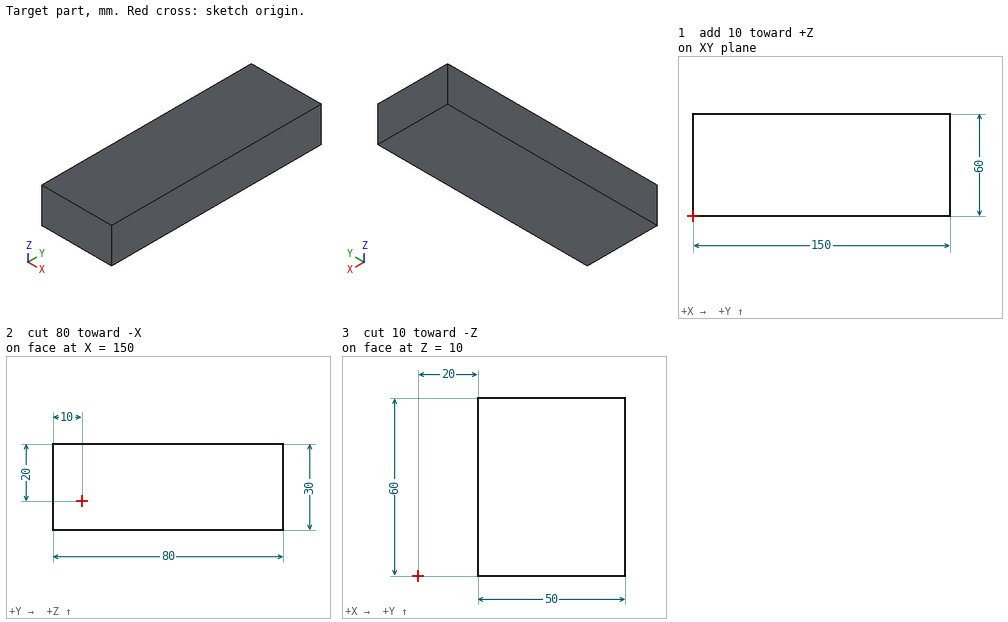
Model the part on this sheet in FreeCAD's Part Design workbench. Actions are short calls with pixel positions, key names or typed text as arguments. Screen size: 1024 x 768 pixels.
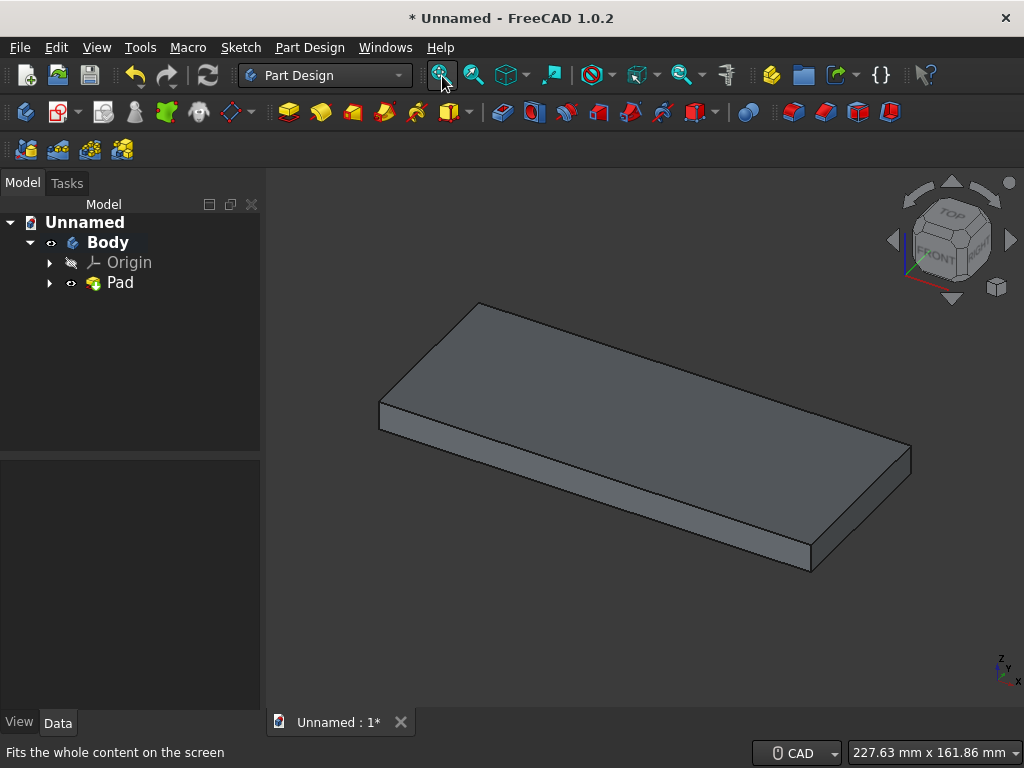
click(890, 480)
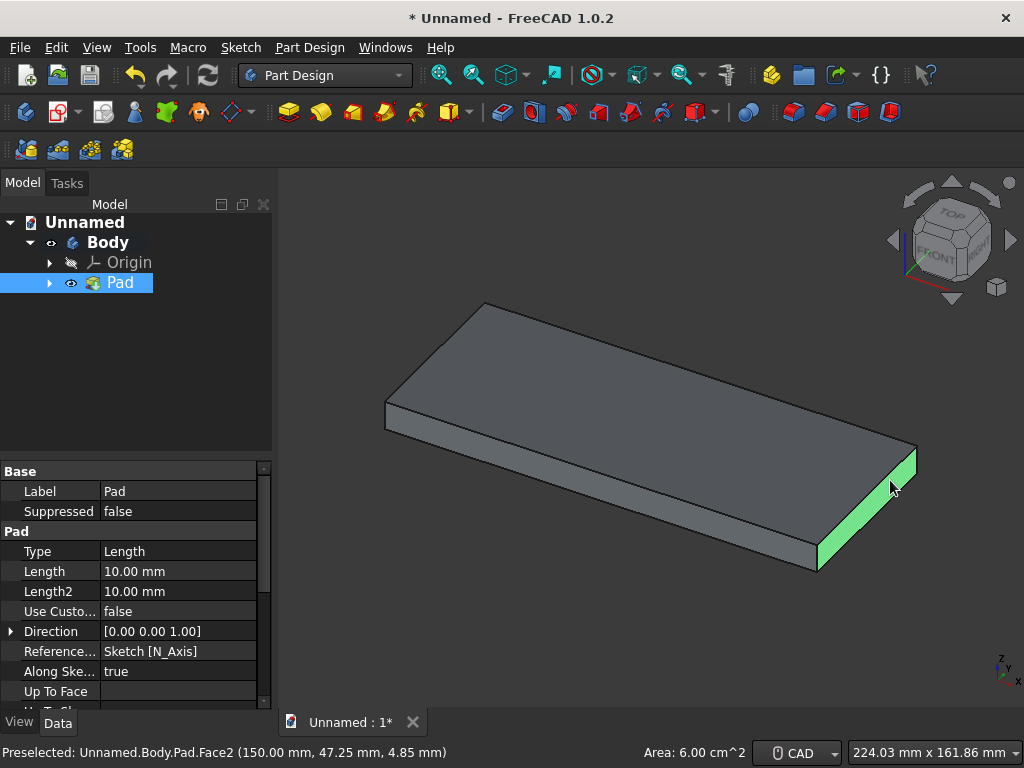
click(58, 112)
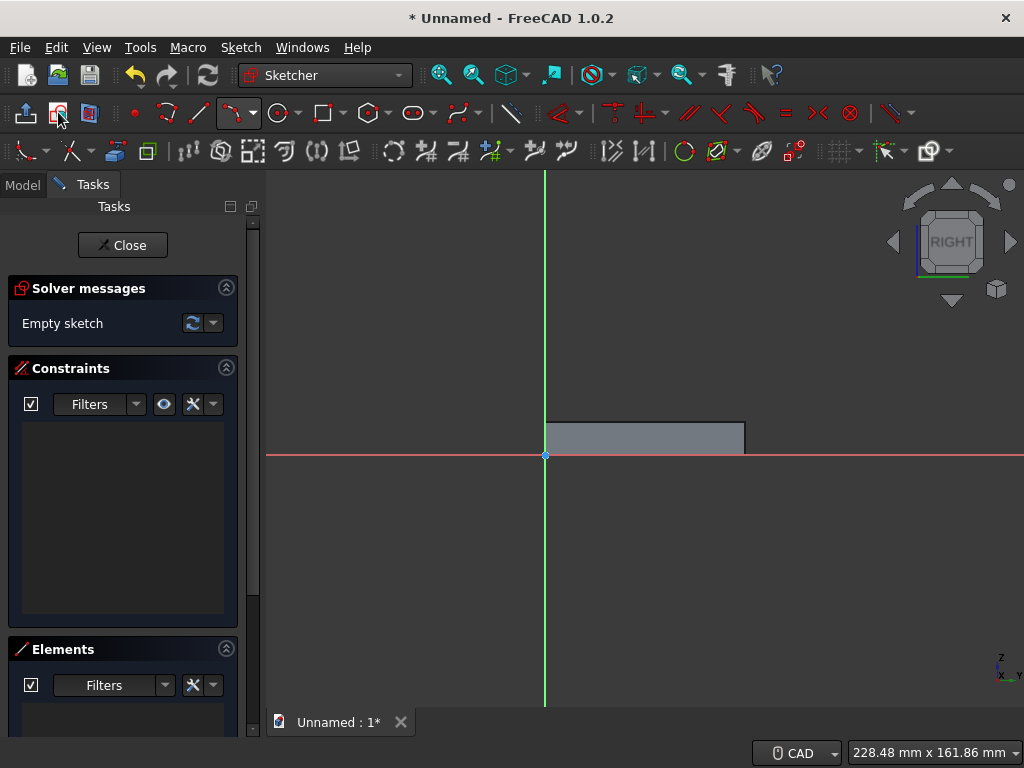
scroll(784, 439, up, 2)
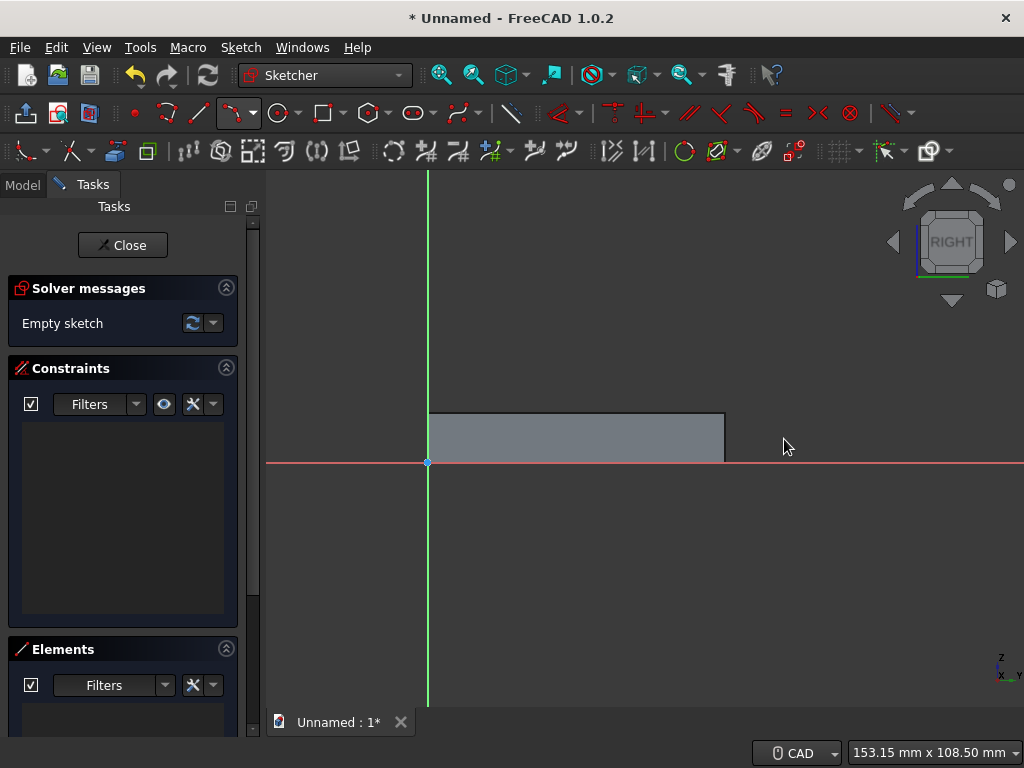
click(324, 114)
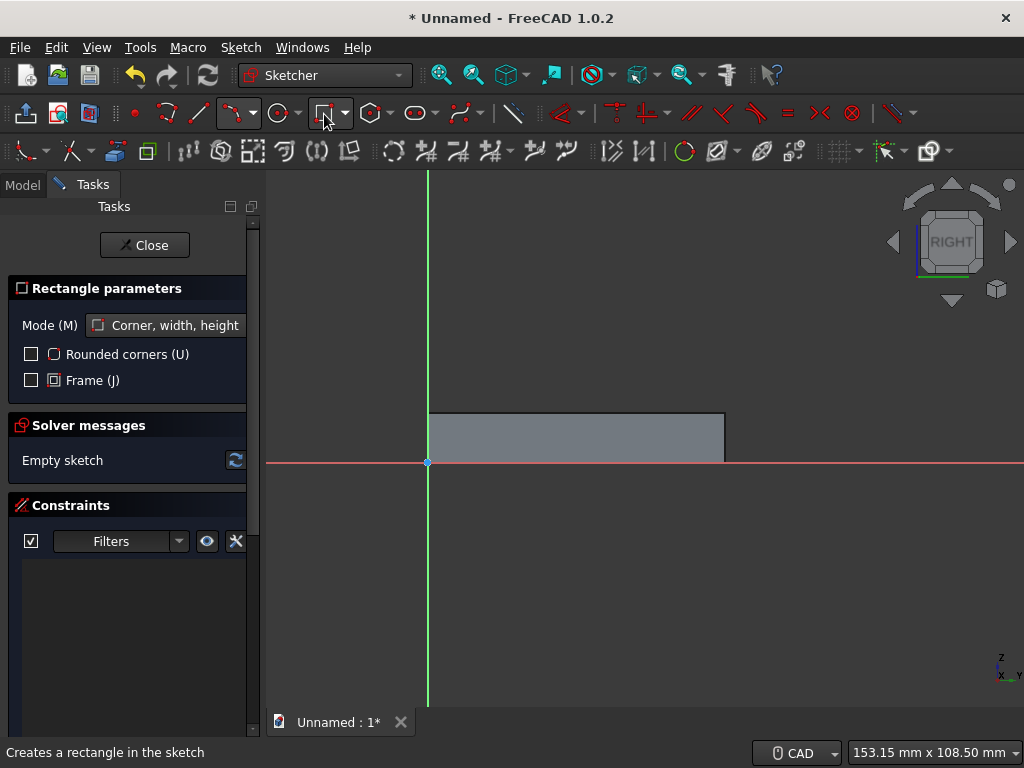
click(378, 364)
move(774, 512)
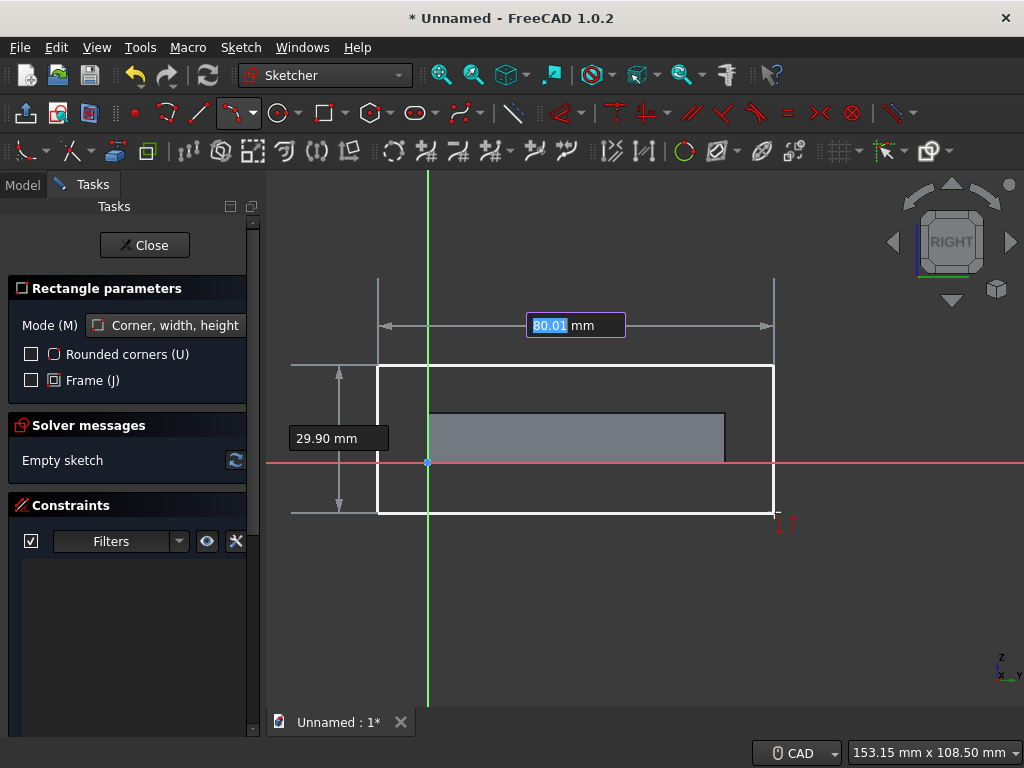
text(80)
key(Tab)
text(30)
key(Return)
key(Escape)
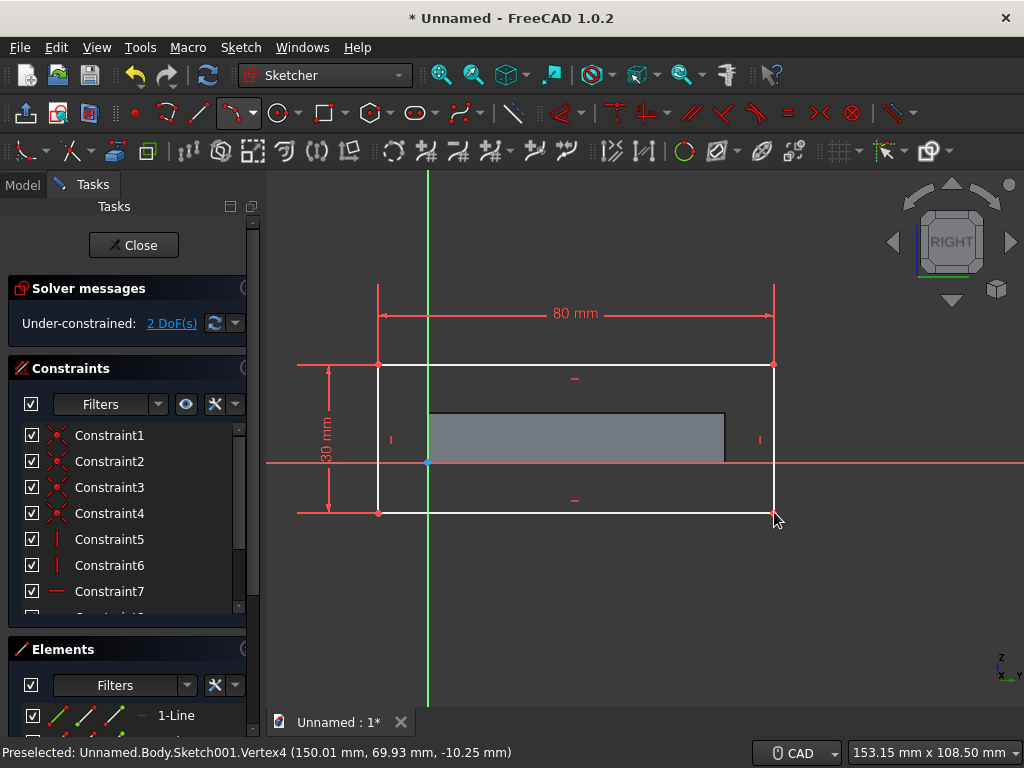
click(560, 114)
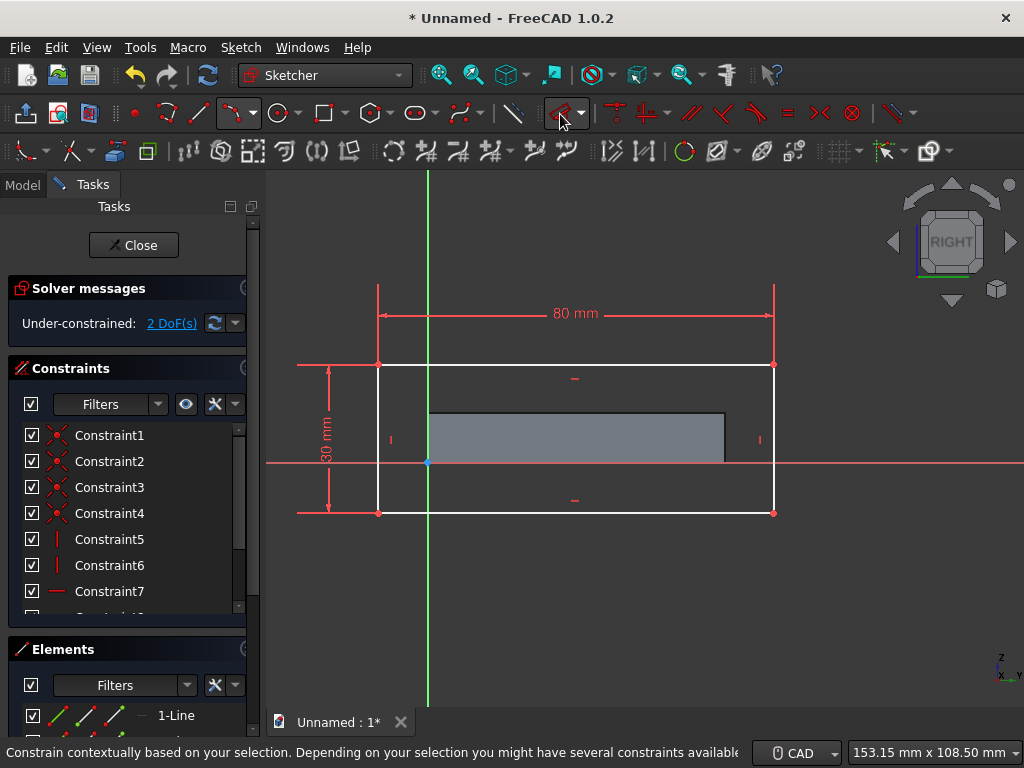
click(378, 365)
click(403, 331)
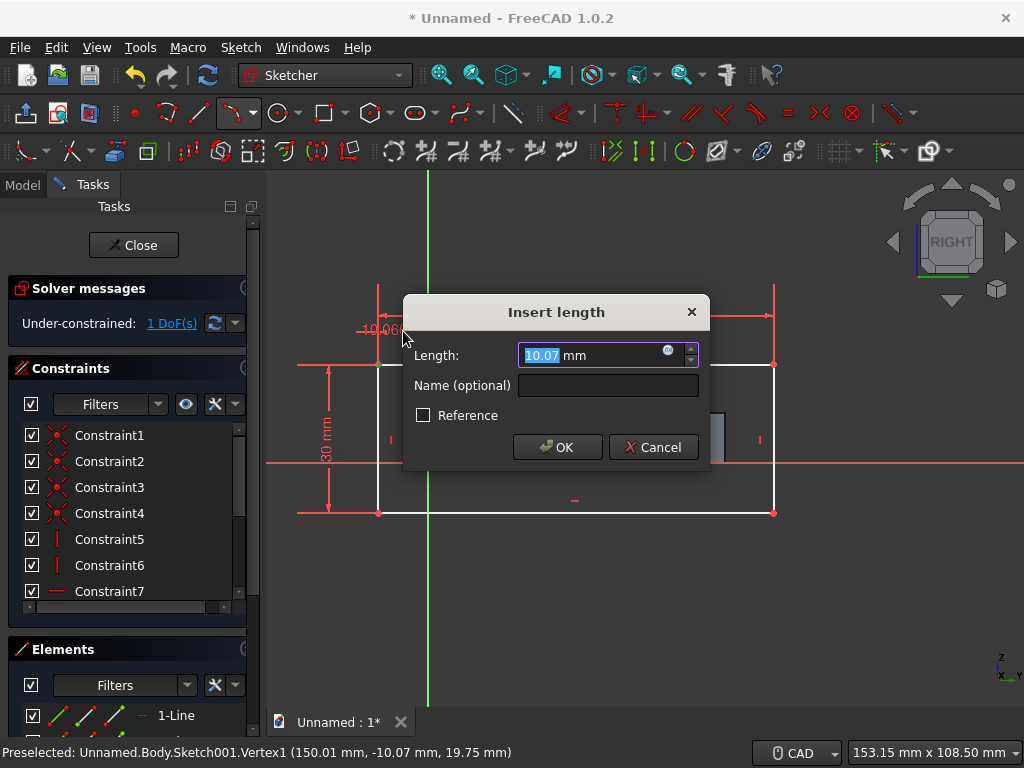
text(10)
key(Return)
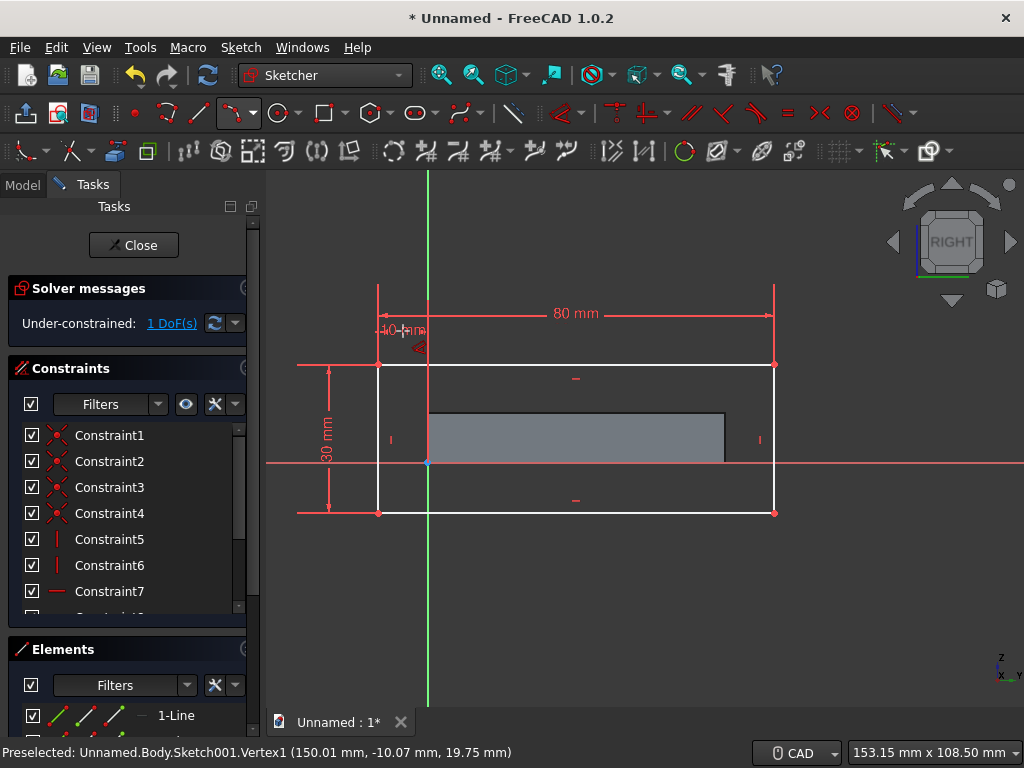
click(378, 365)
click(344, 414)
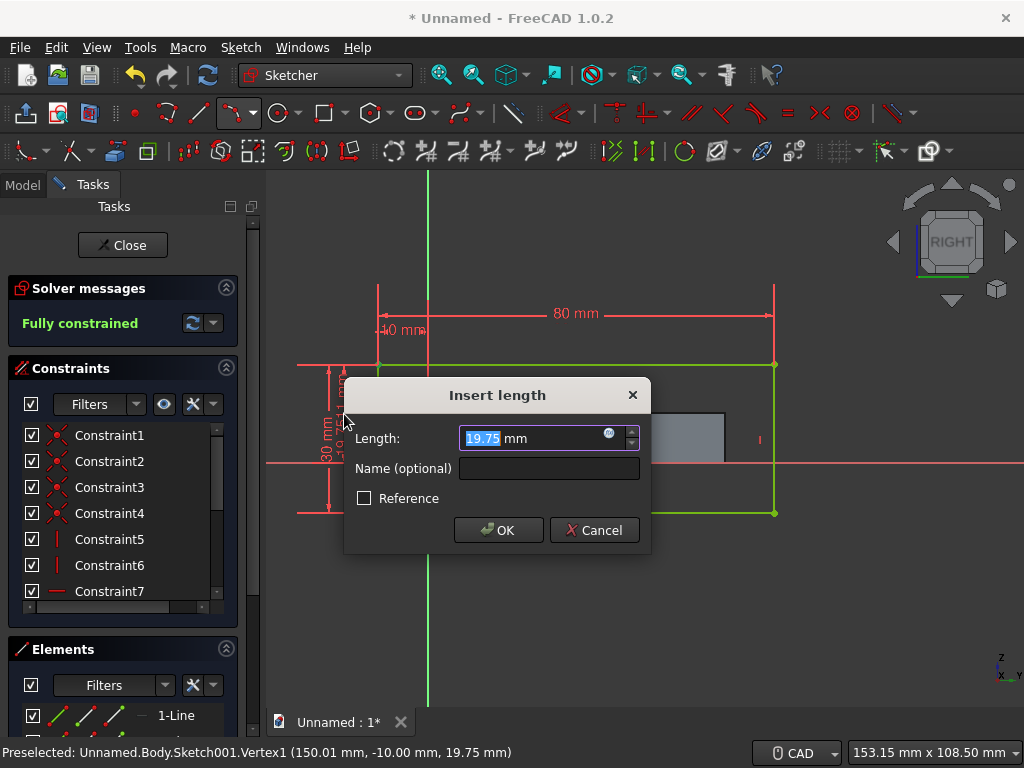
text(20)
key(Return)
key(Escape)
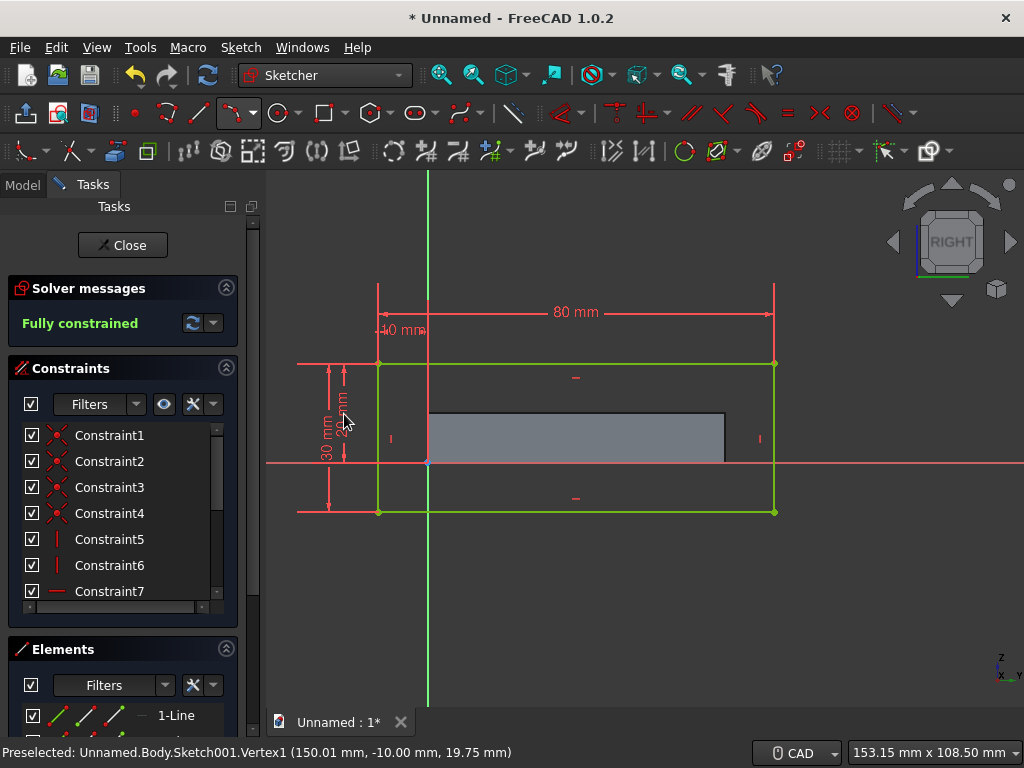
click(123, 245)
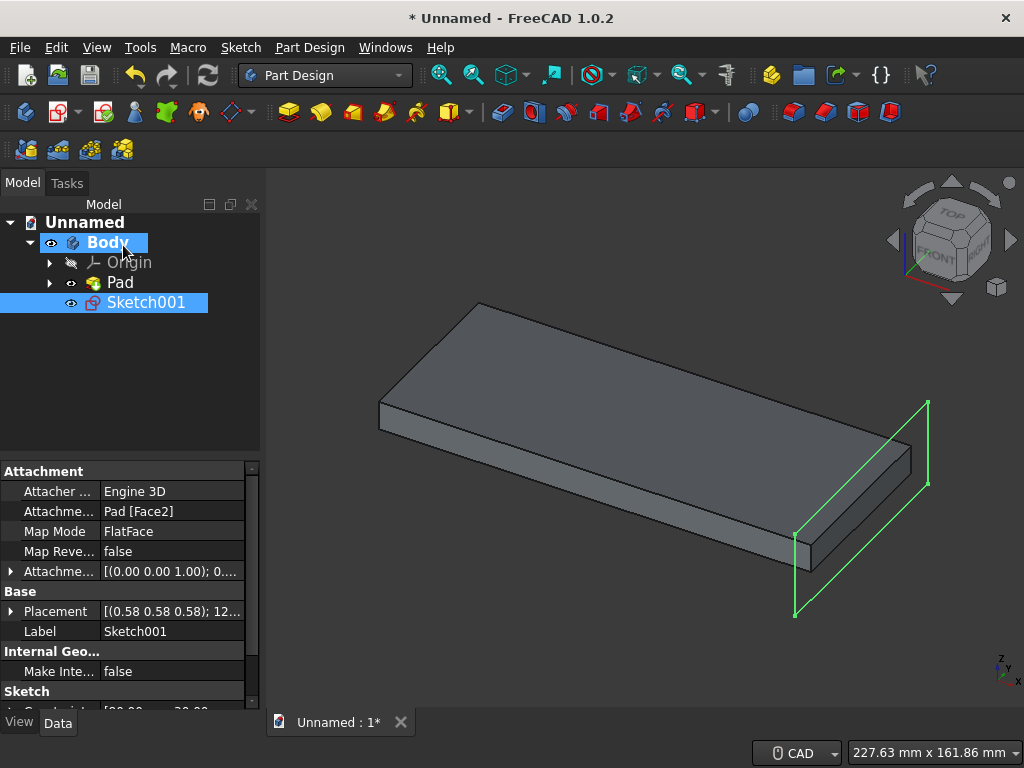
click(504, 112)